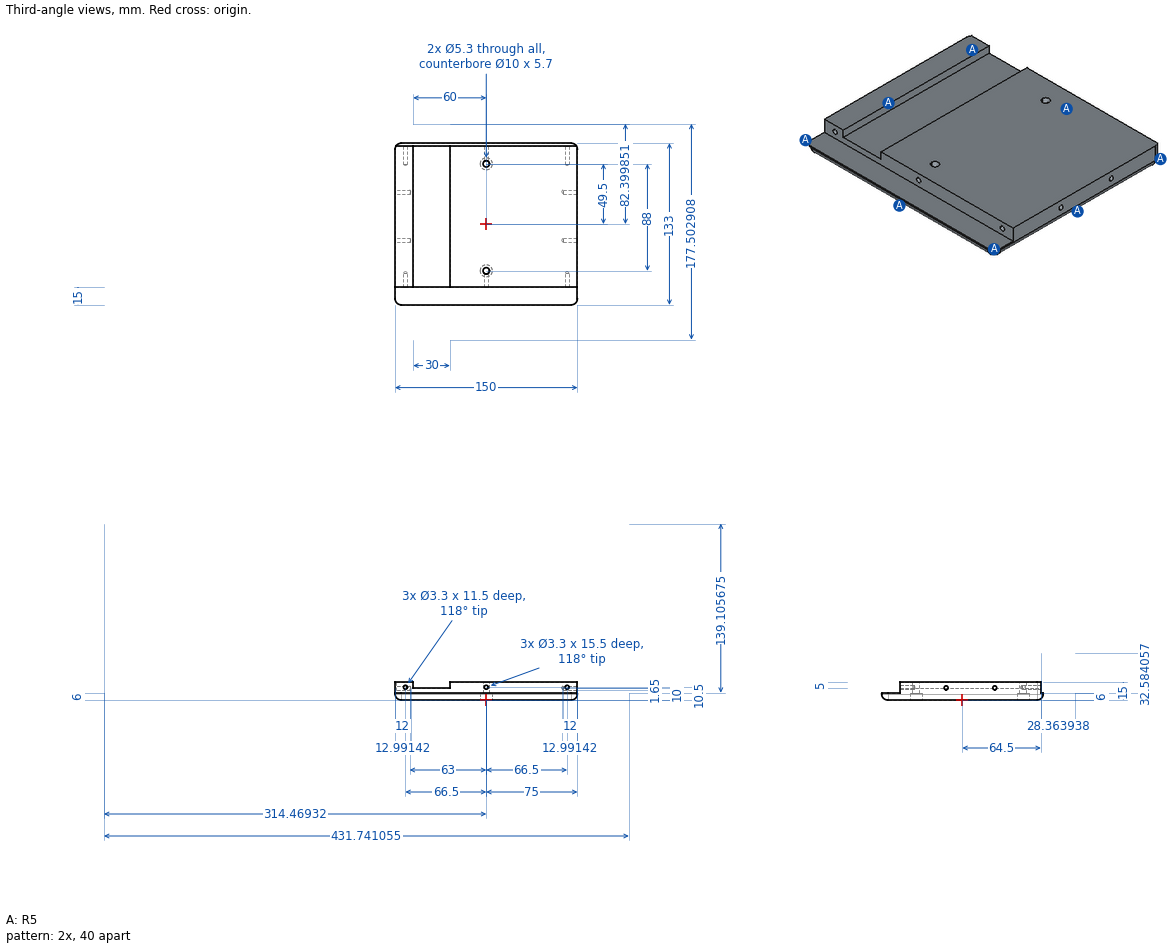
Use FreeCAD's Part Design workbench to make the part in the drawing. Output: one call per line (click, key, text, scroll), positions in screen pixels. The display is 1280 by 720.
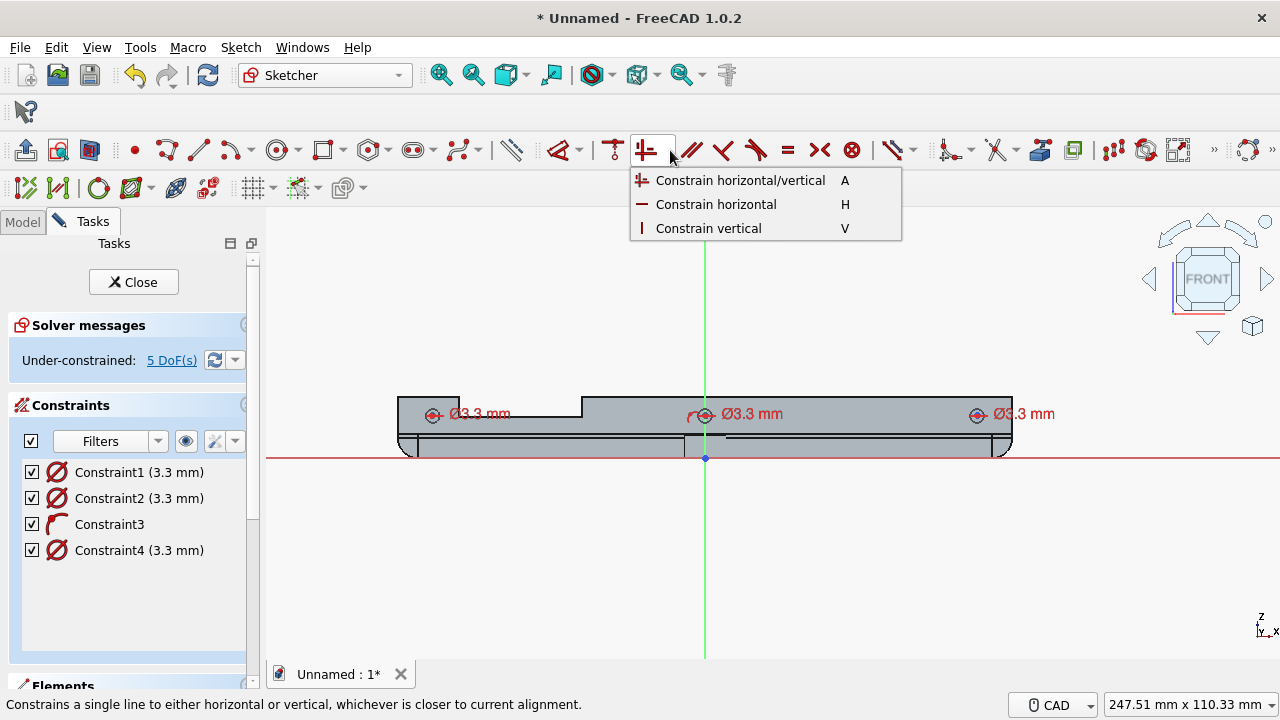
click(766, 204)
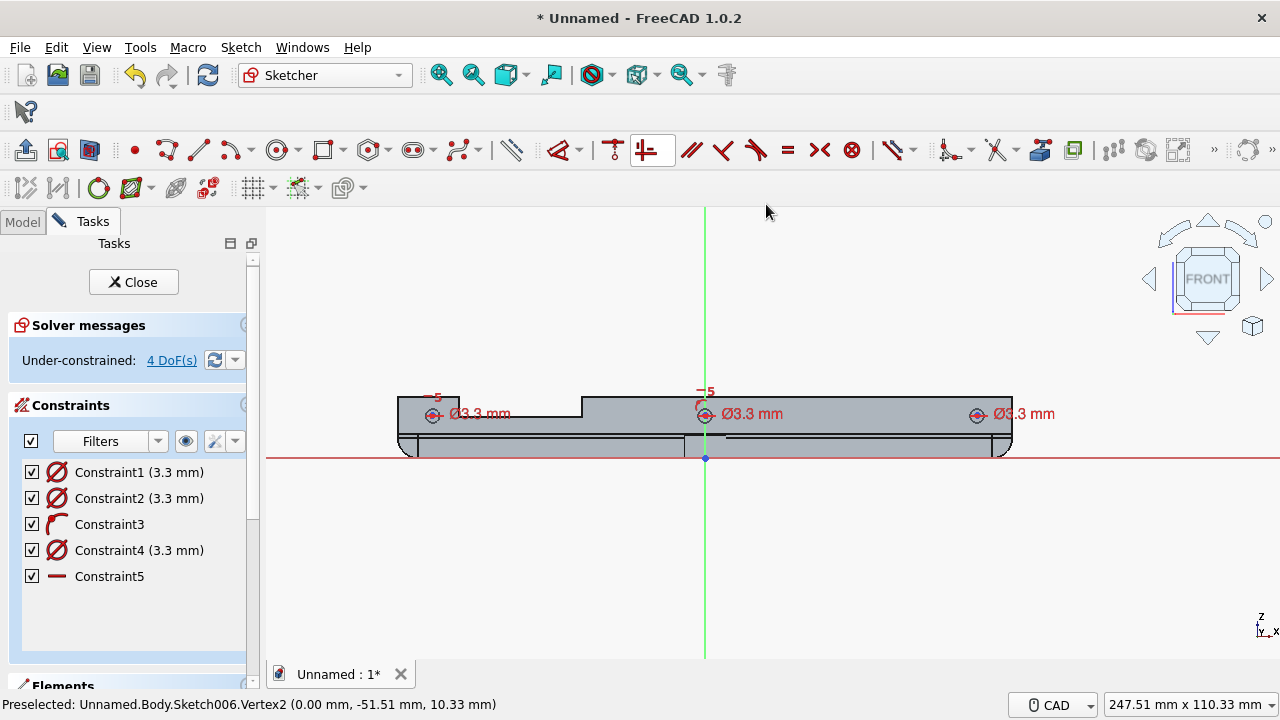
click(705, 416)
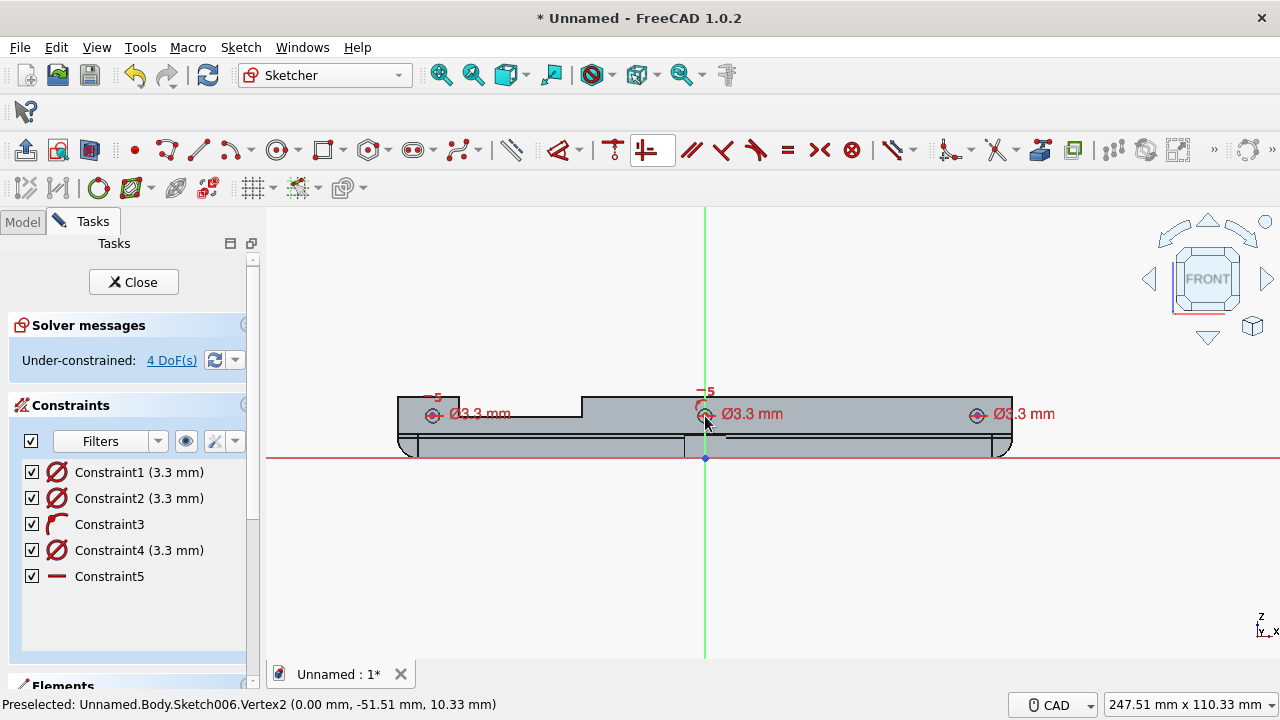
click(977, 416)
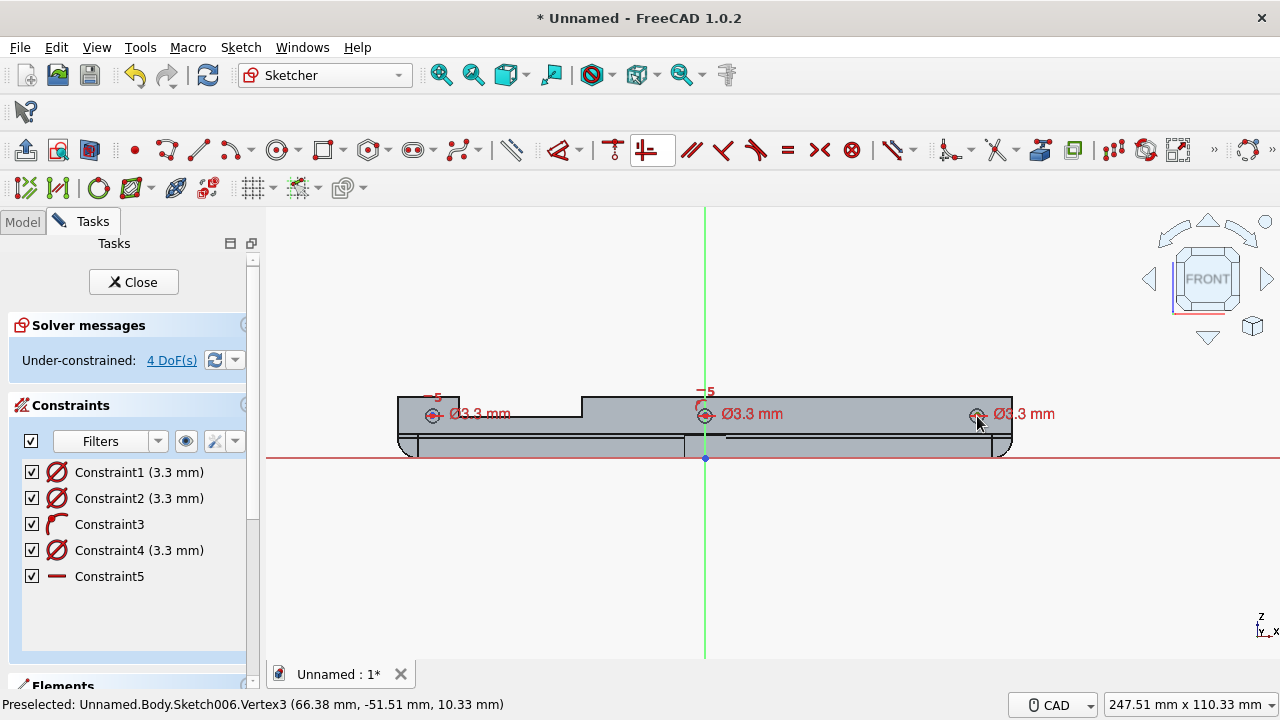
key(h)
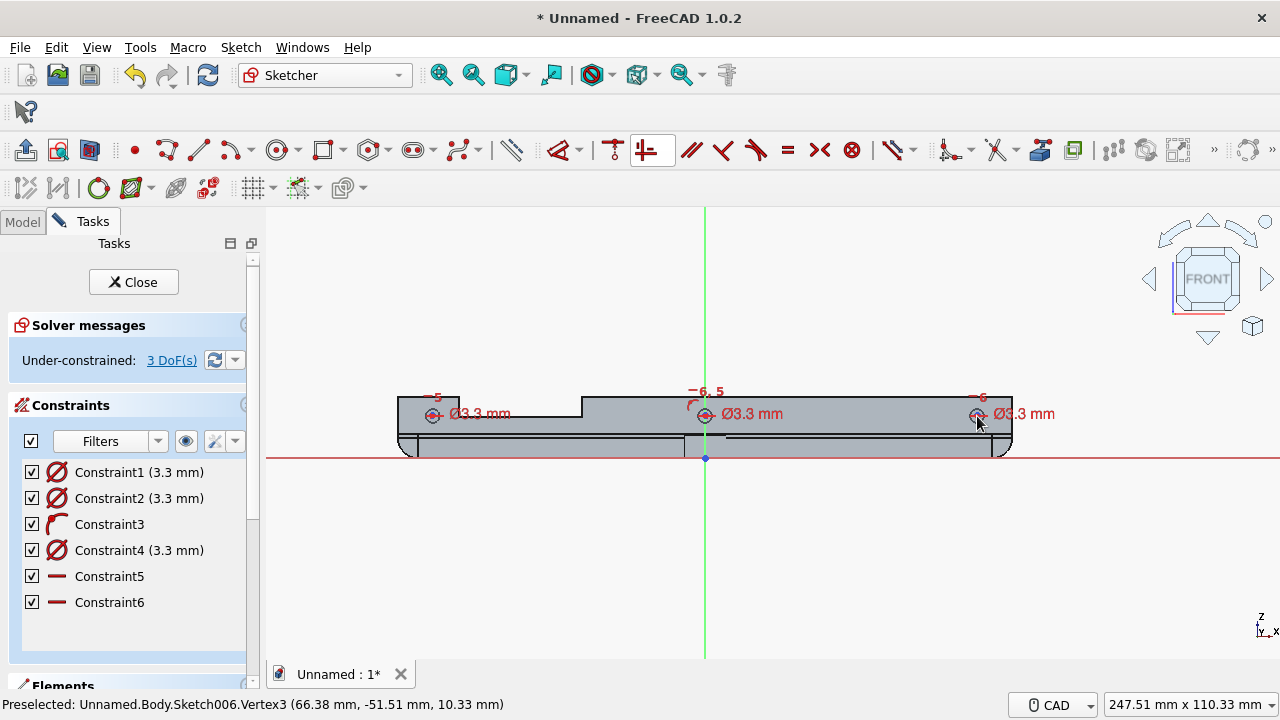
click(558, 150)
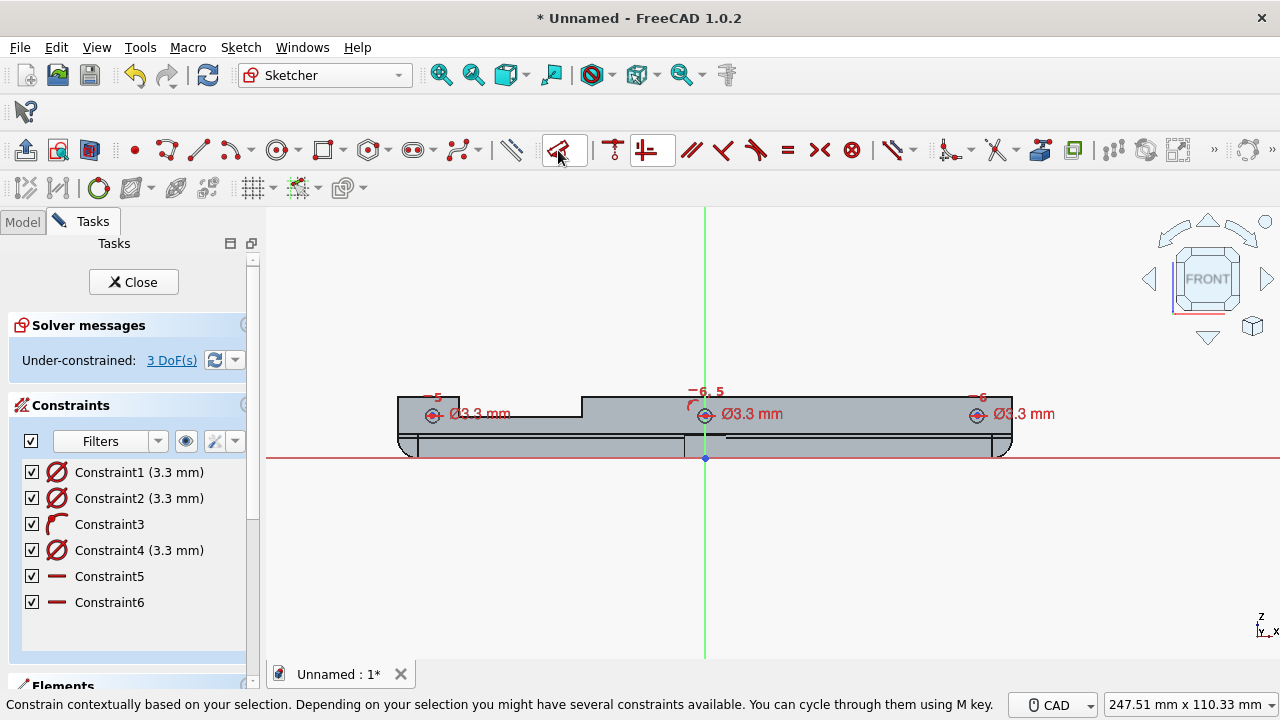
click(433, 416)
click(569, 492)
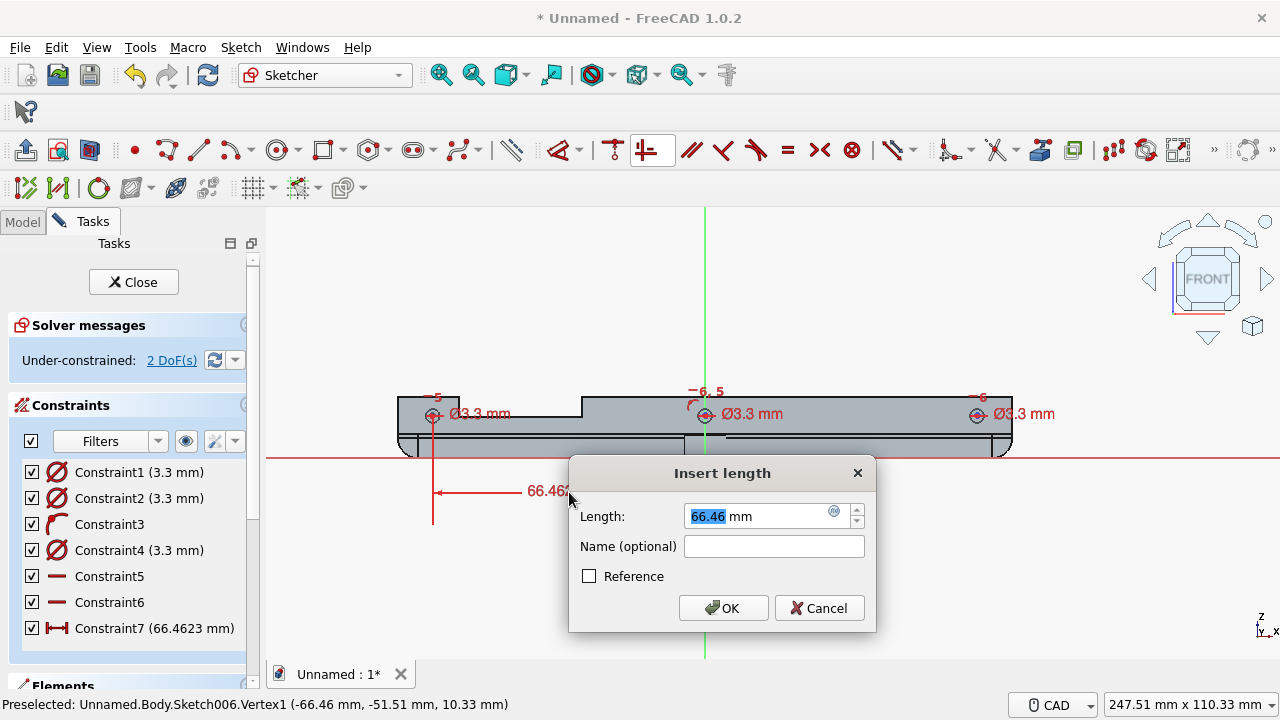
text(66.5)
key(Return)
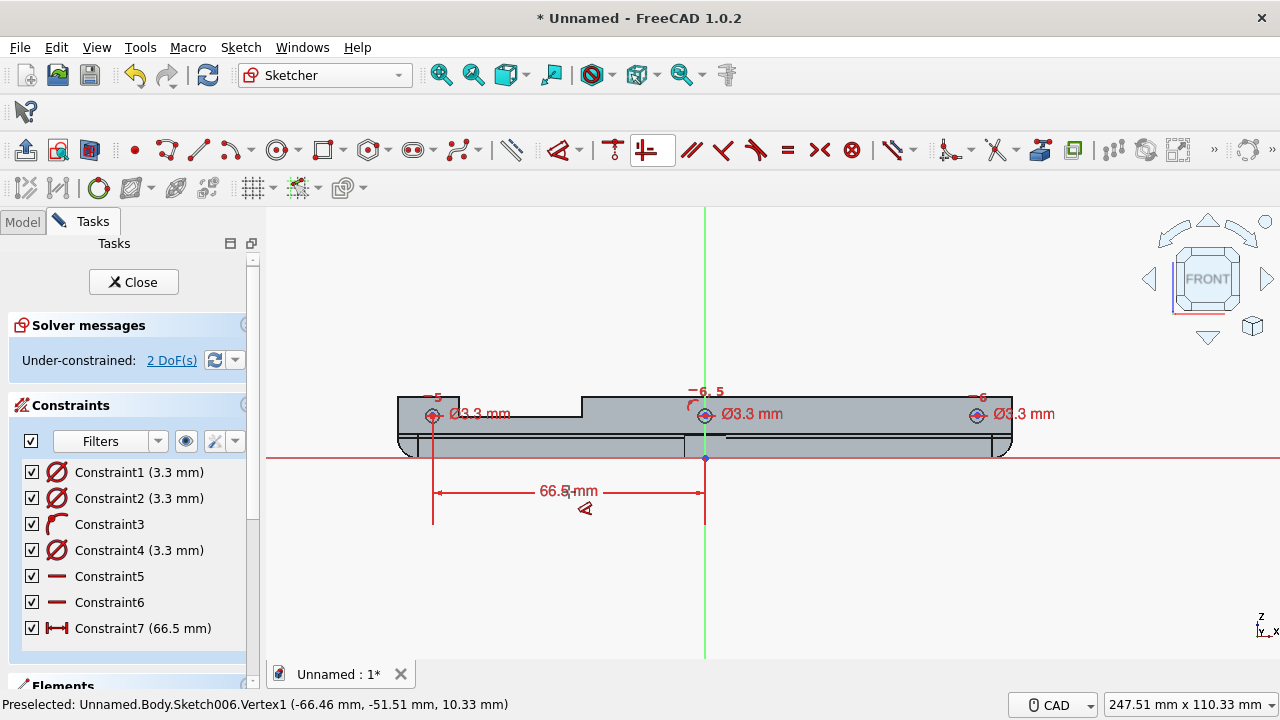
click(433, 416)
click(399, 437)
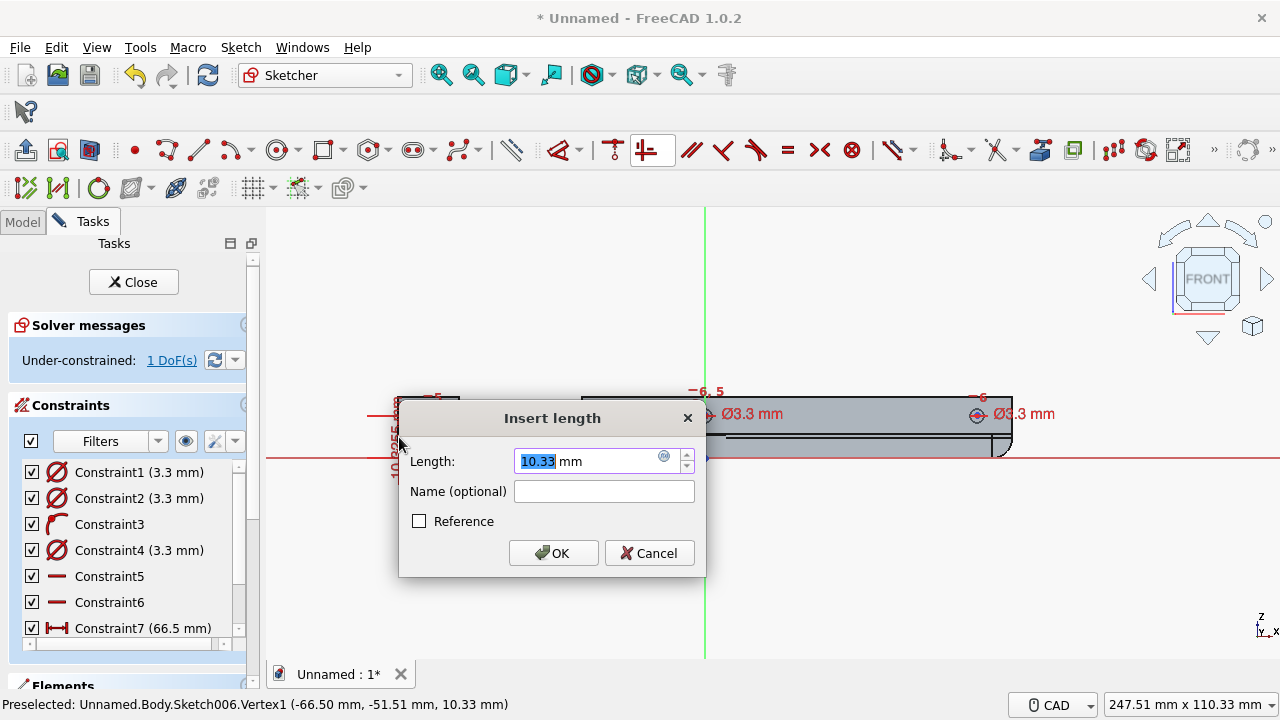
text(10.5)
key(Return)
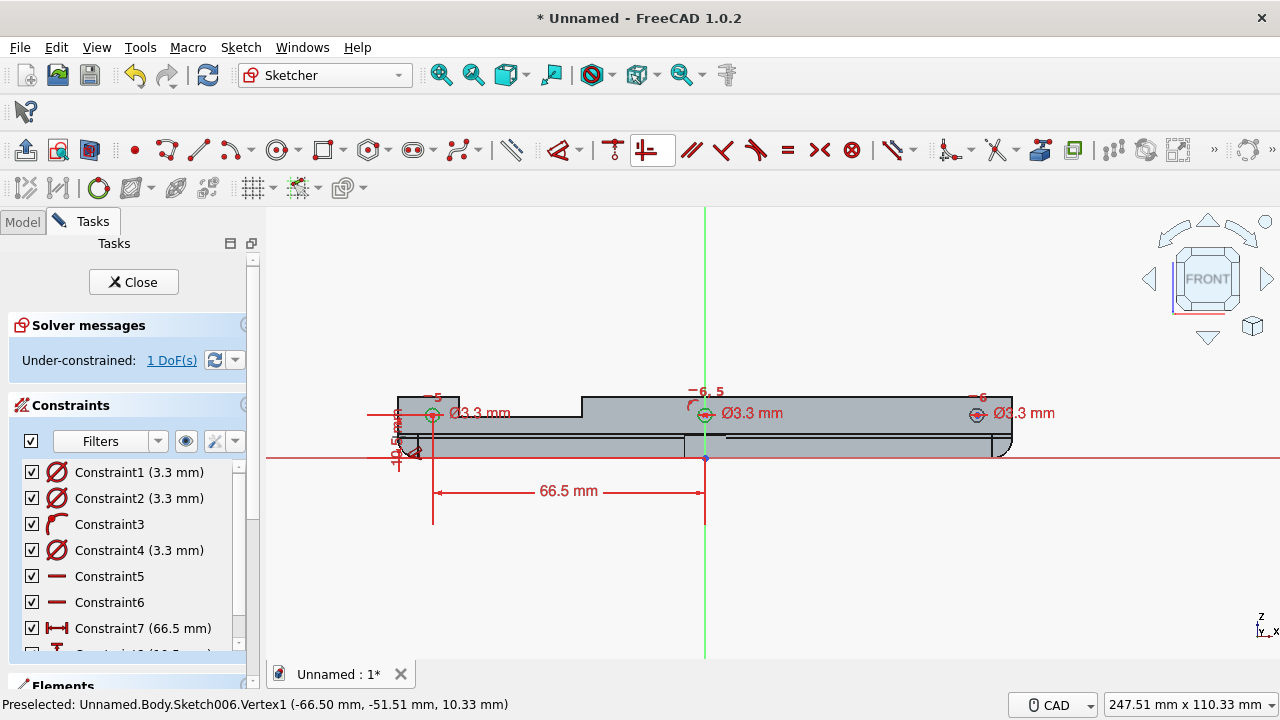
click(977, 415)
click(841, 492)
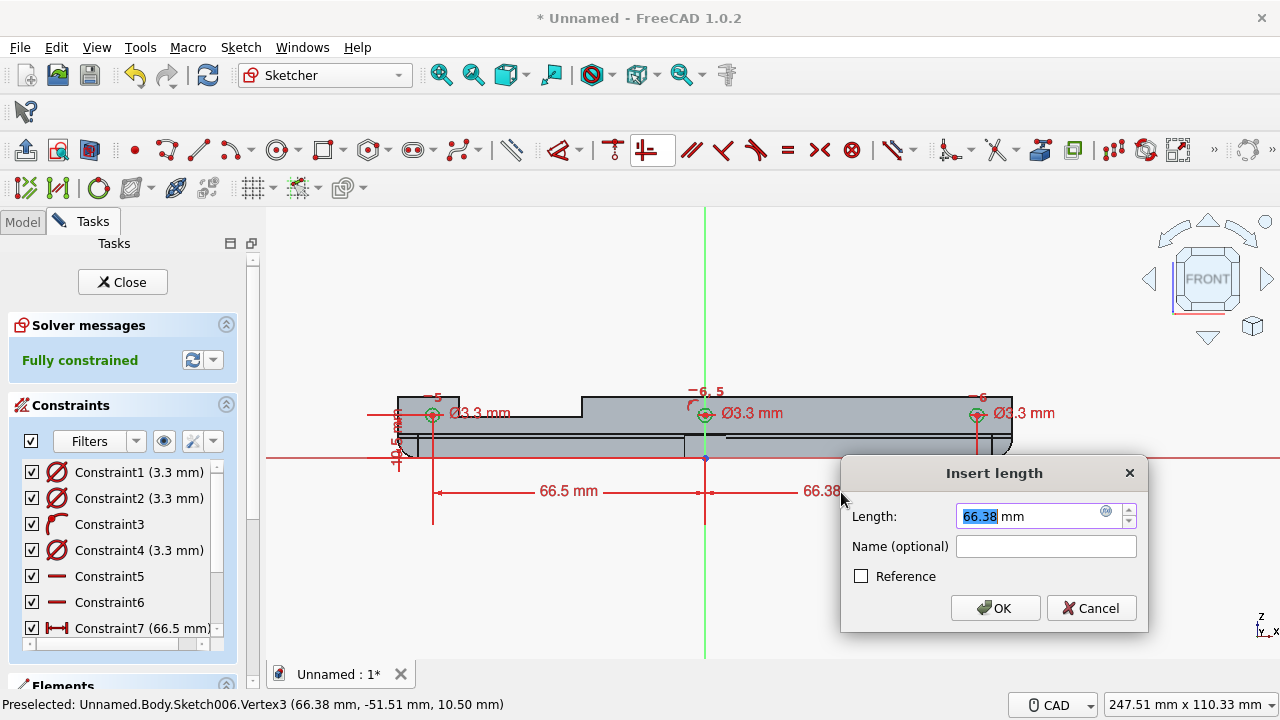
text(66.5)
key(Return)
key(Escape)